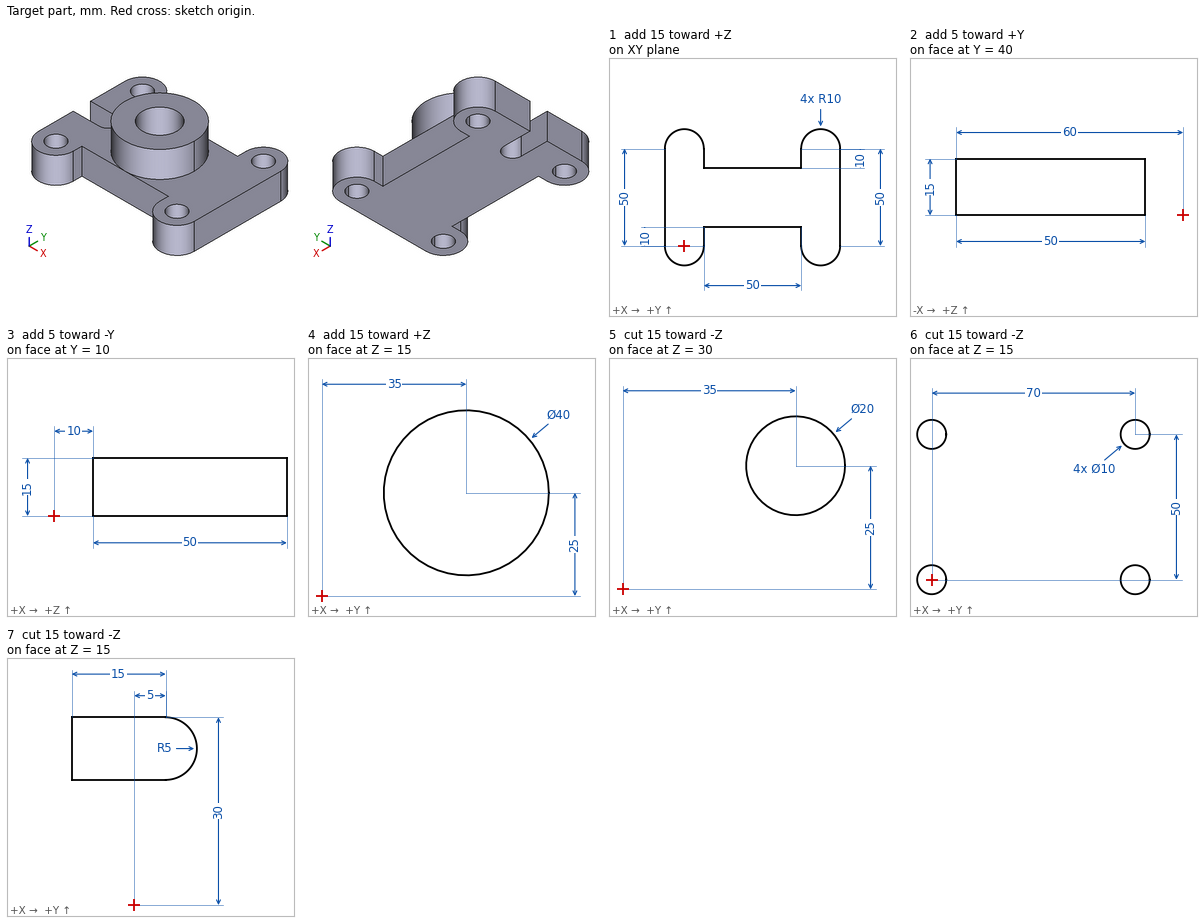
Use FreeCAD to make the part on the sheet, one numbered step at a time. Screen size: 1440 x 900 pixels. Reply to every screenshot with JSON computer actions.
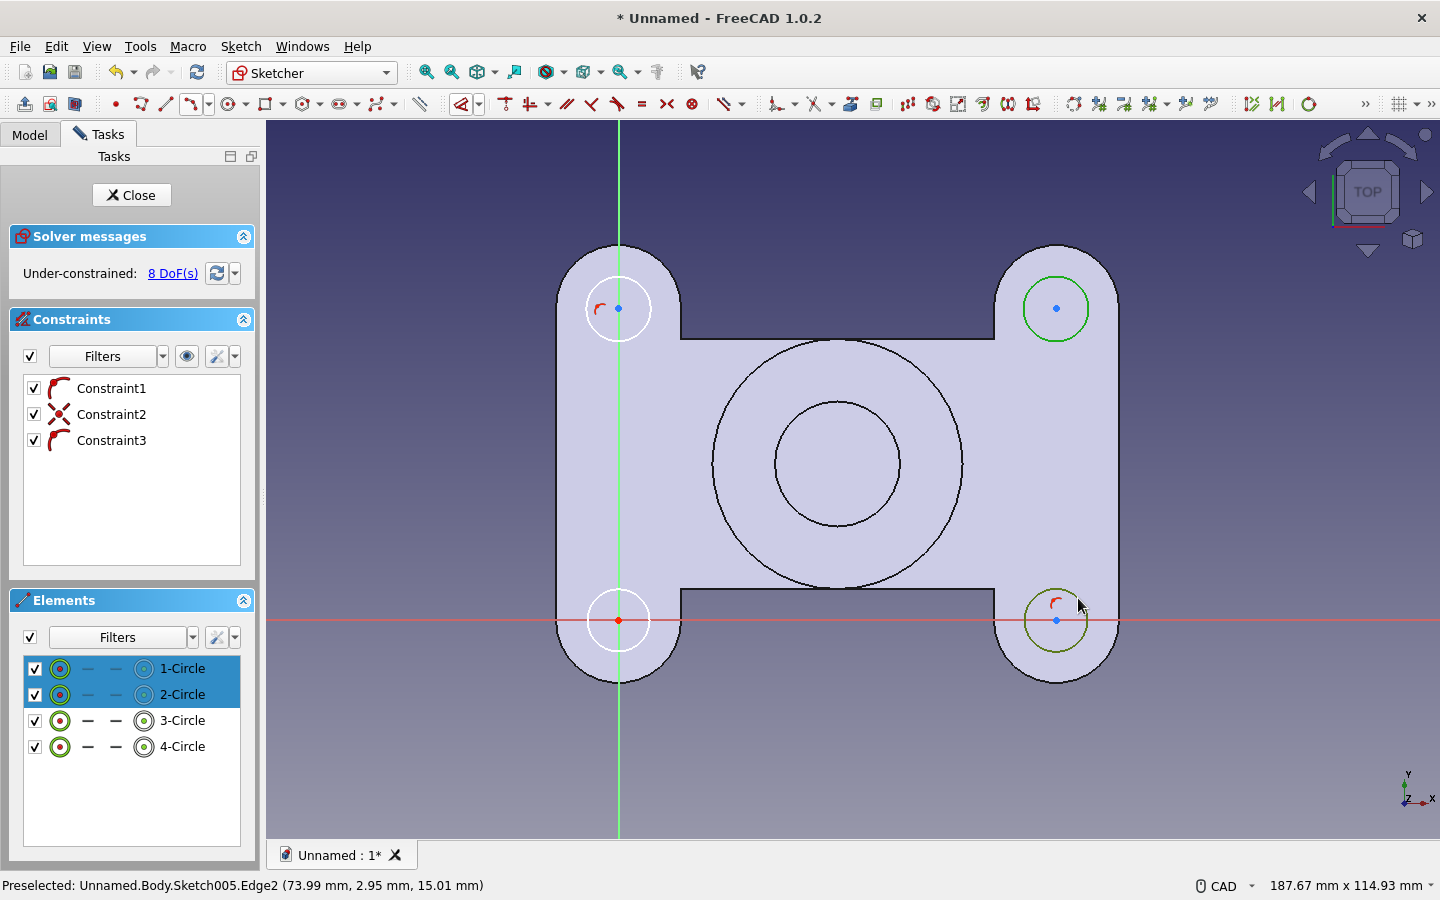
{"action": "left_click", "coordinate": [640, 598]}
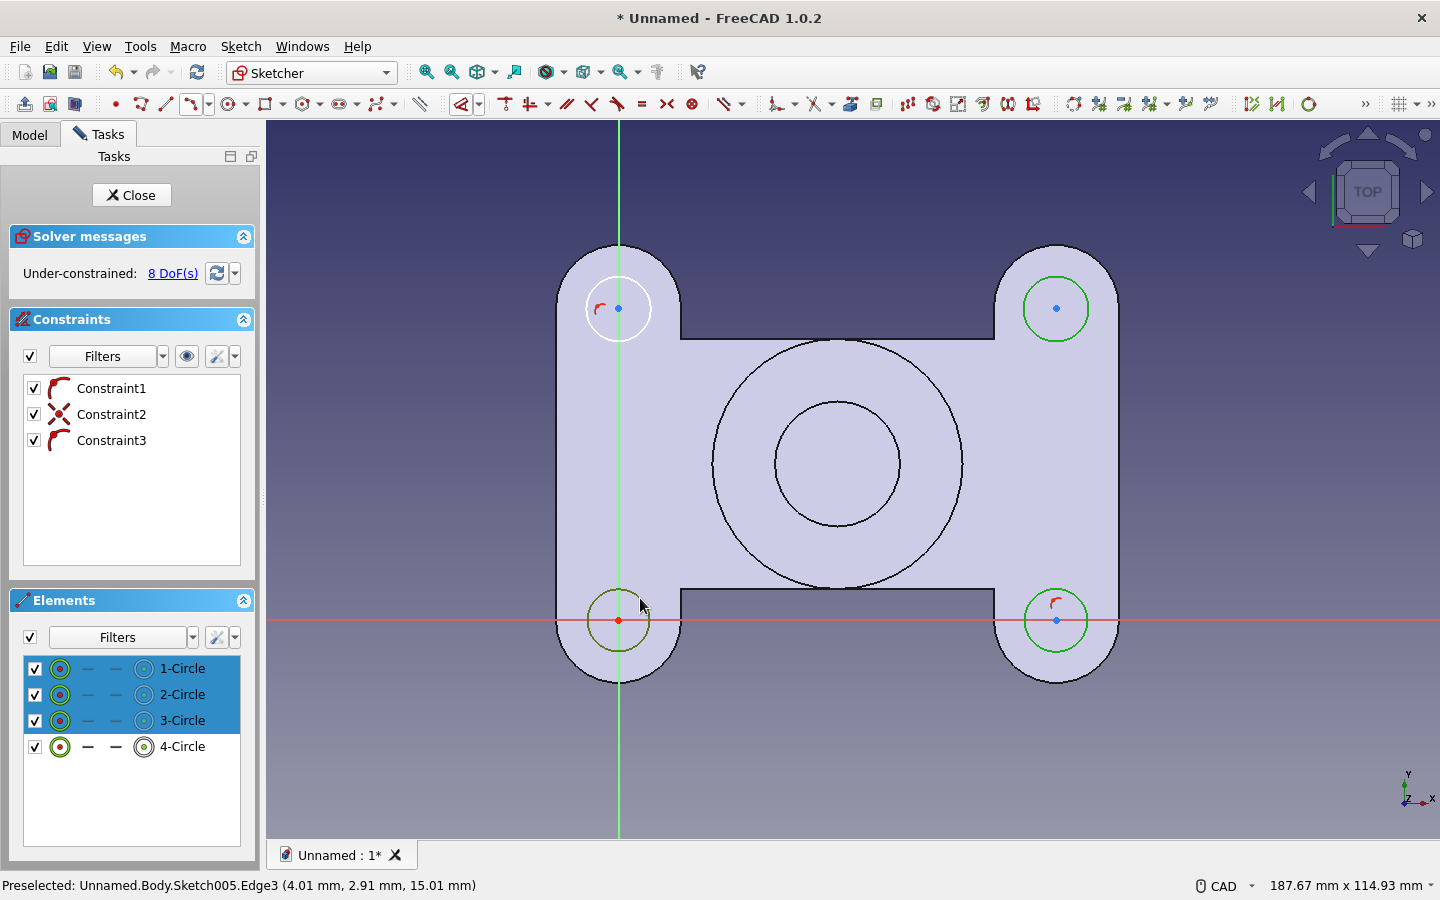
{"action": "left_click", "coordinate": [641, 286]}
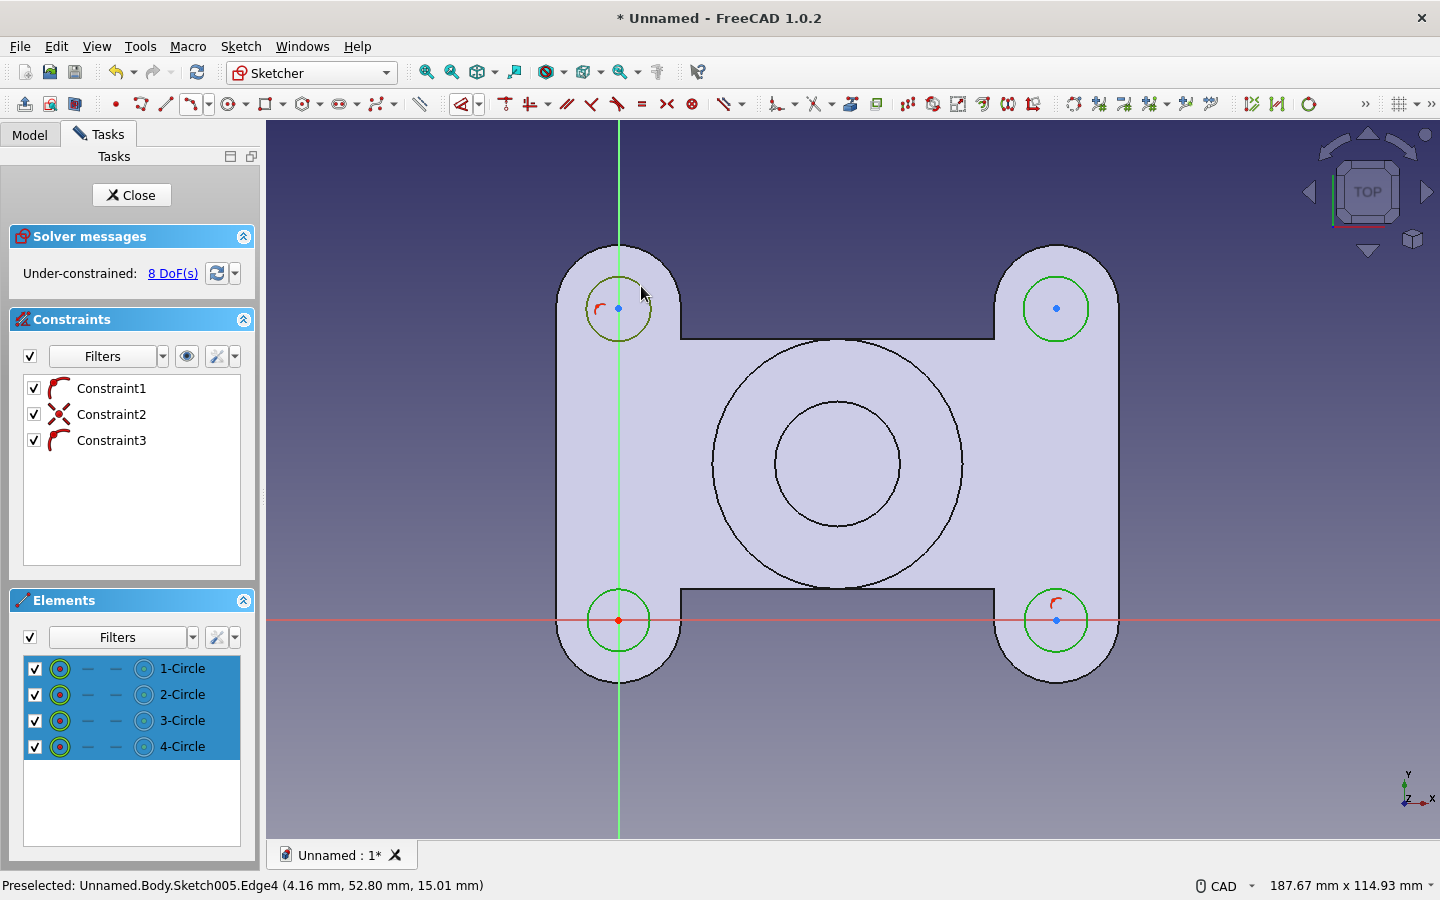
{"action": "key", "text": "e"}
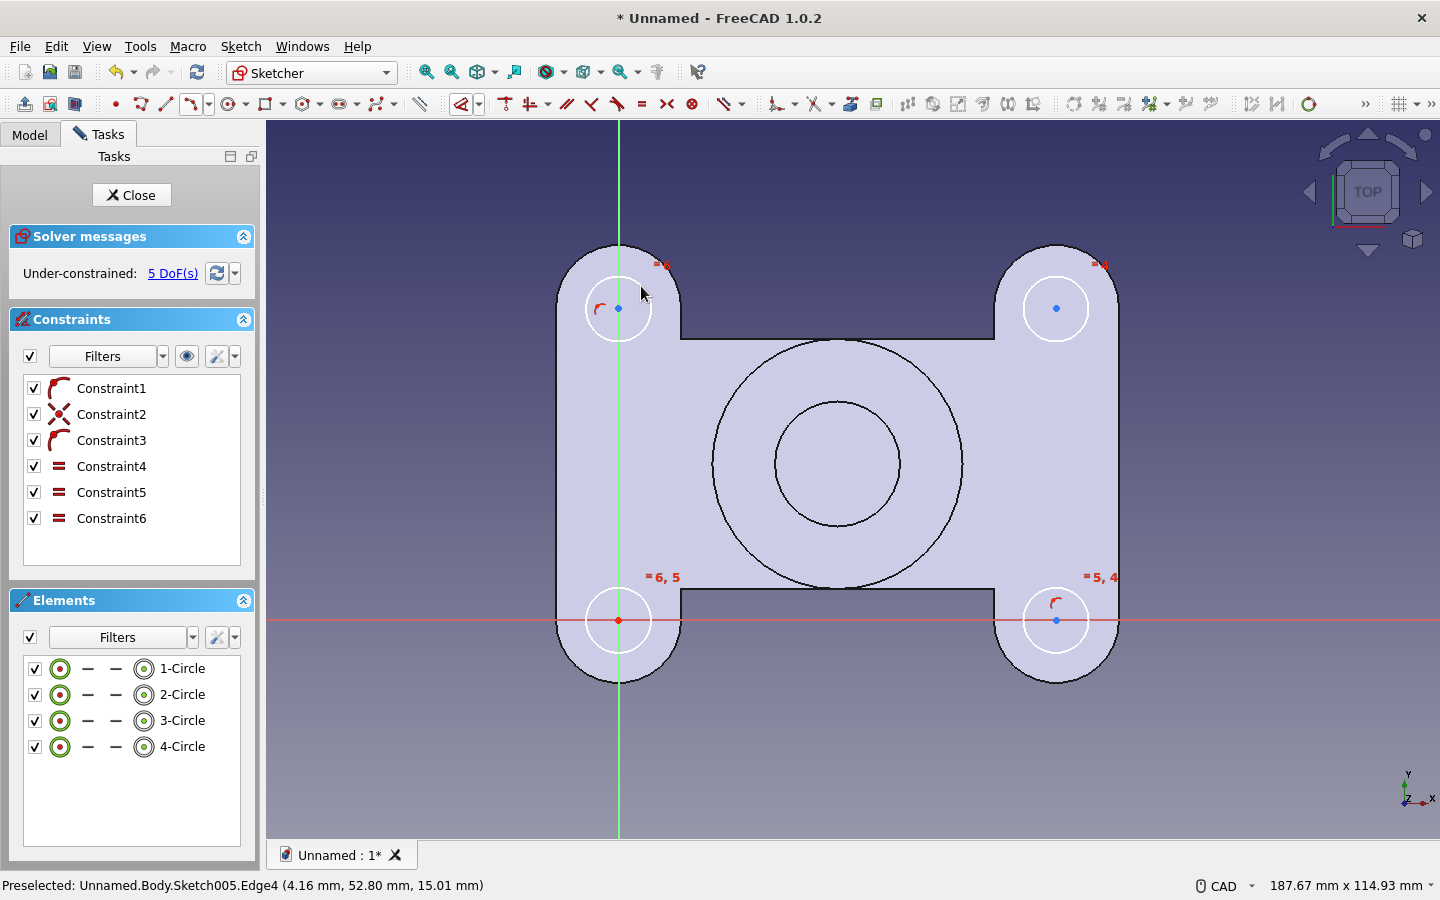
{"action": "left_click", "coordinate": [1056, 309]}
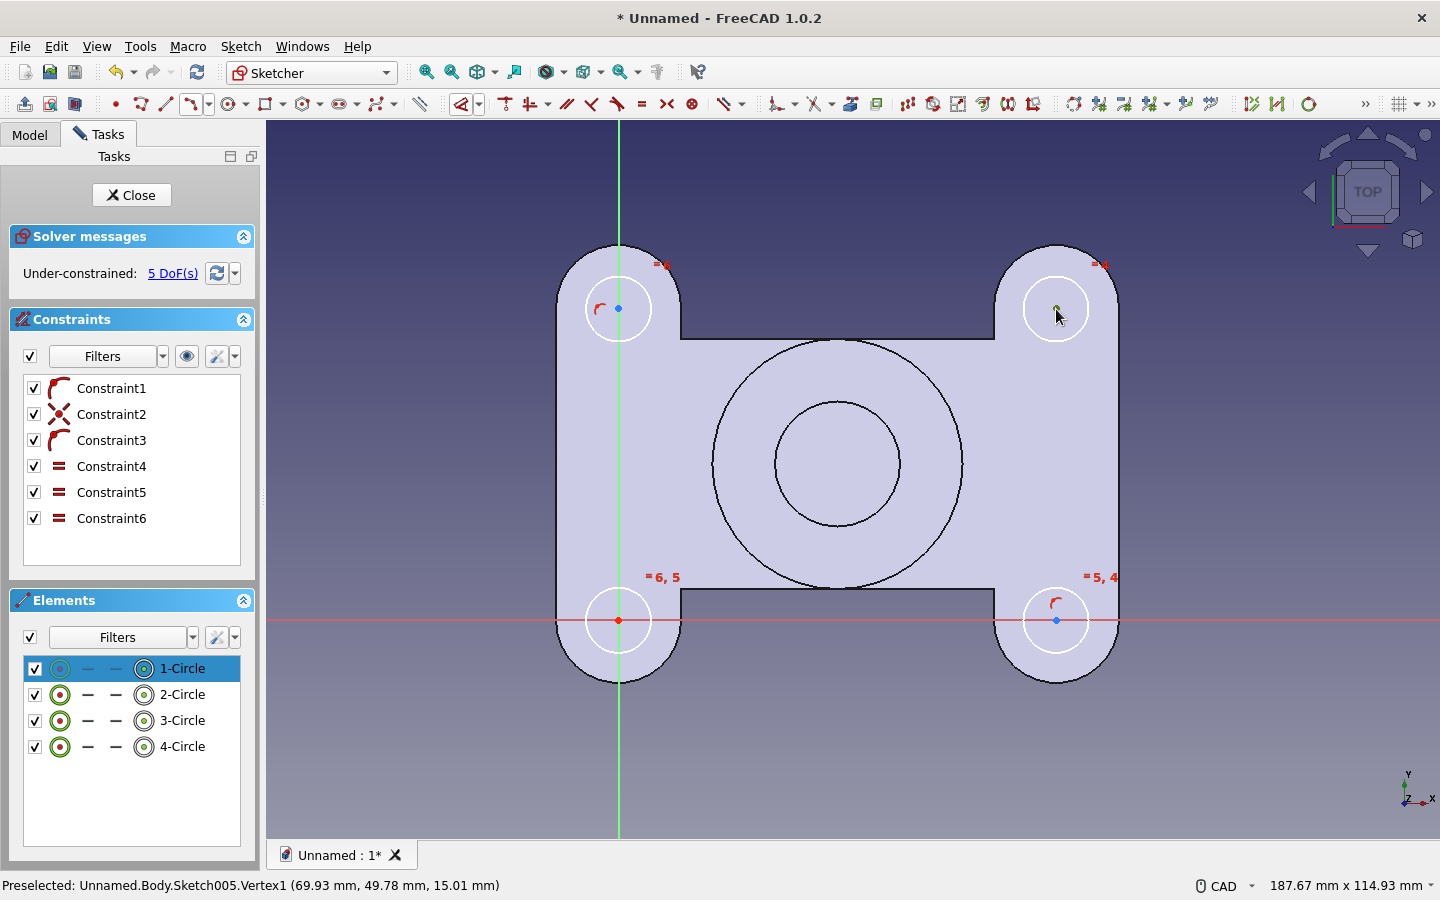
{"action": "left_click", "coordinate": [1056, 620]}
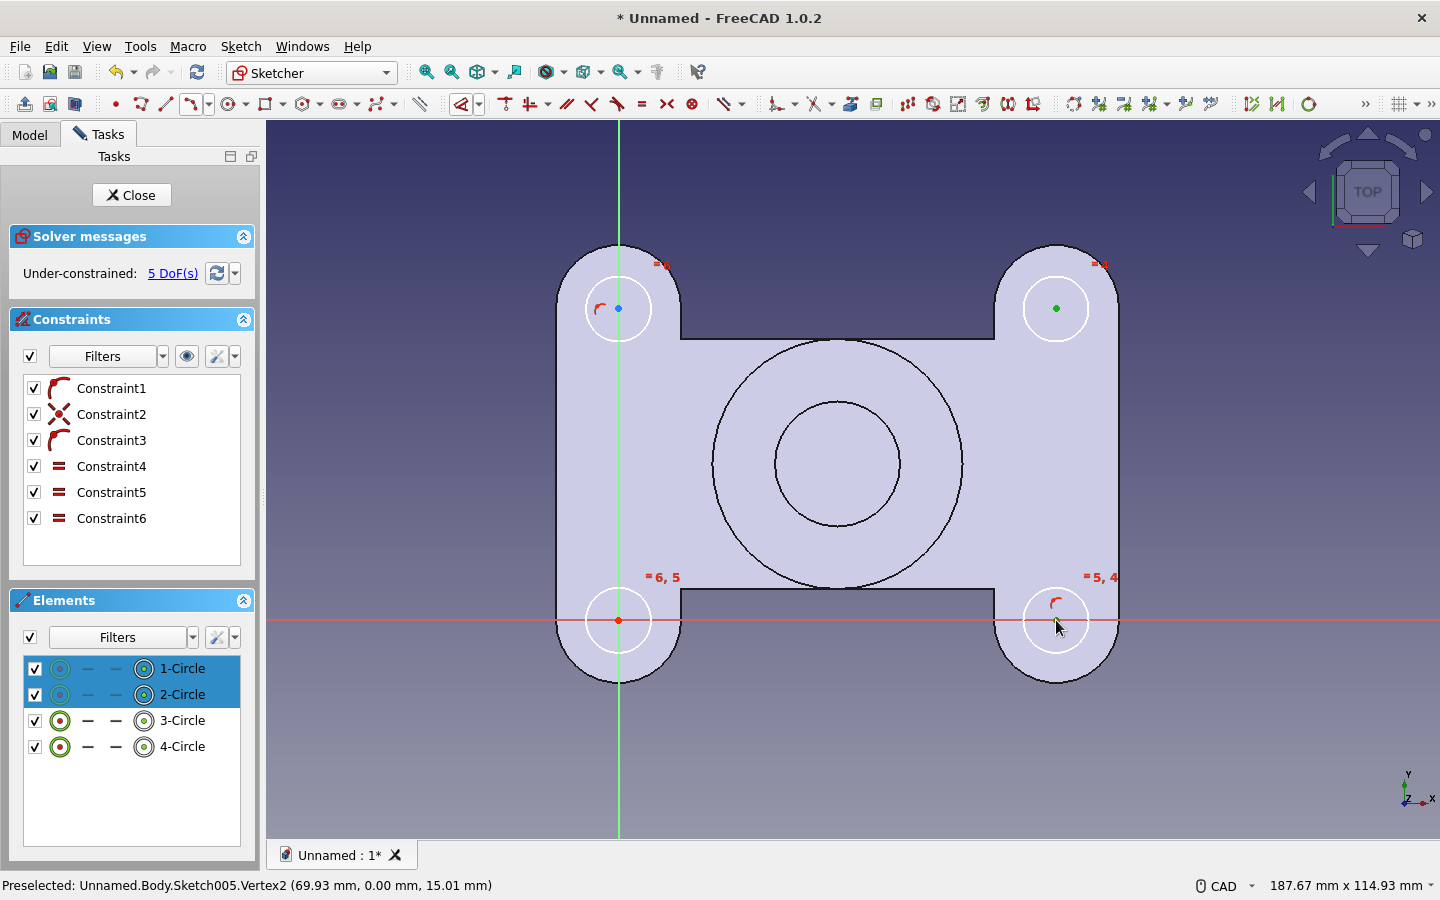
{"action": "left_click", "coordinate": [548, 104]}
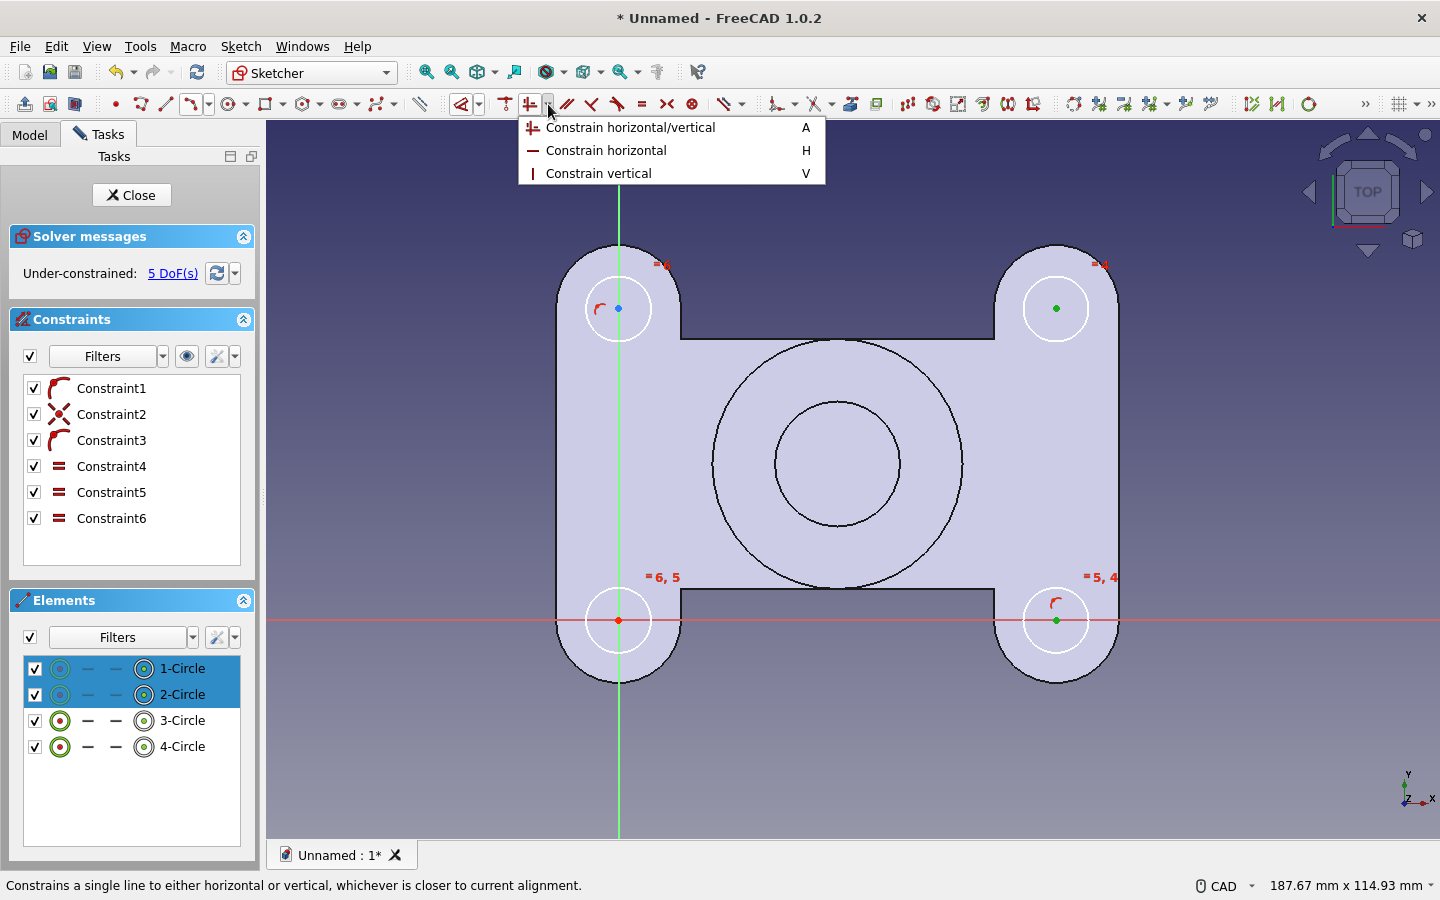
{"action": "left_click", "coordinate": [672, 174]}